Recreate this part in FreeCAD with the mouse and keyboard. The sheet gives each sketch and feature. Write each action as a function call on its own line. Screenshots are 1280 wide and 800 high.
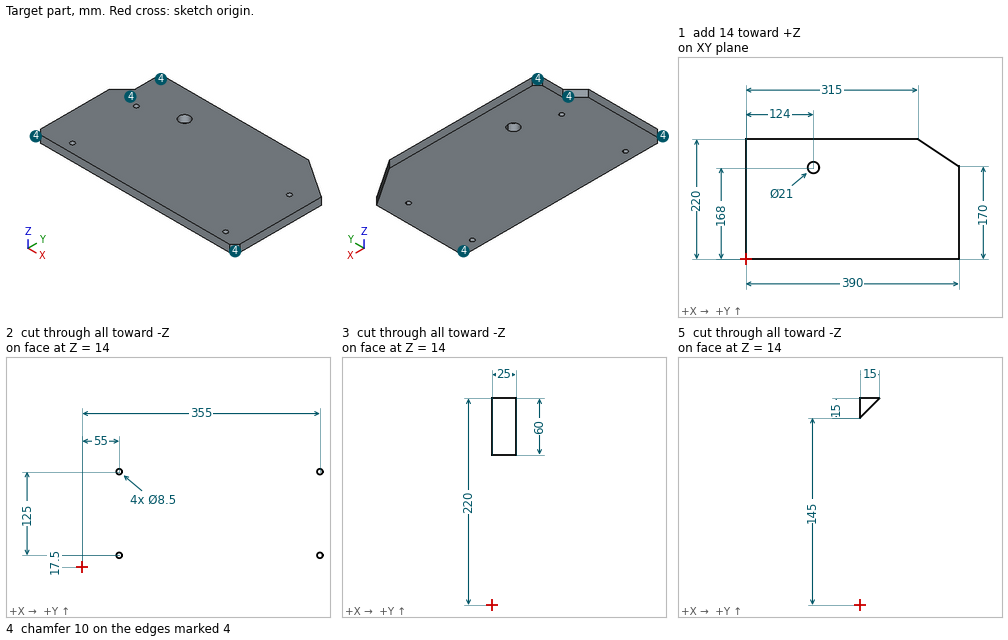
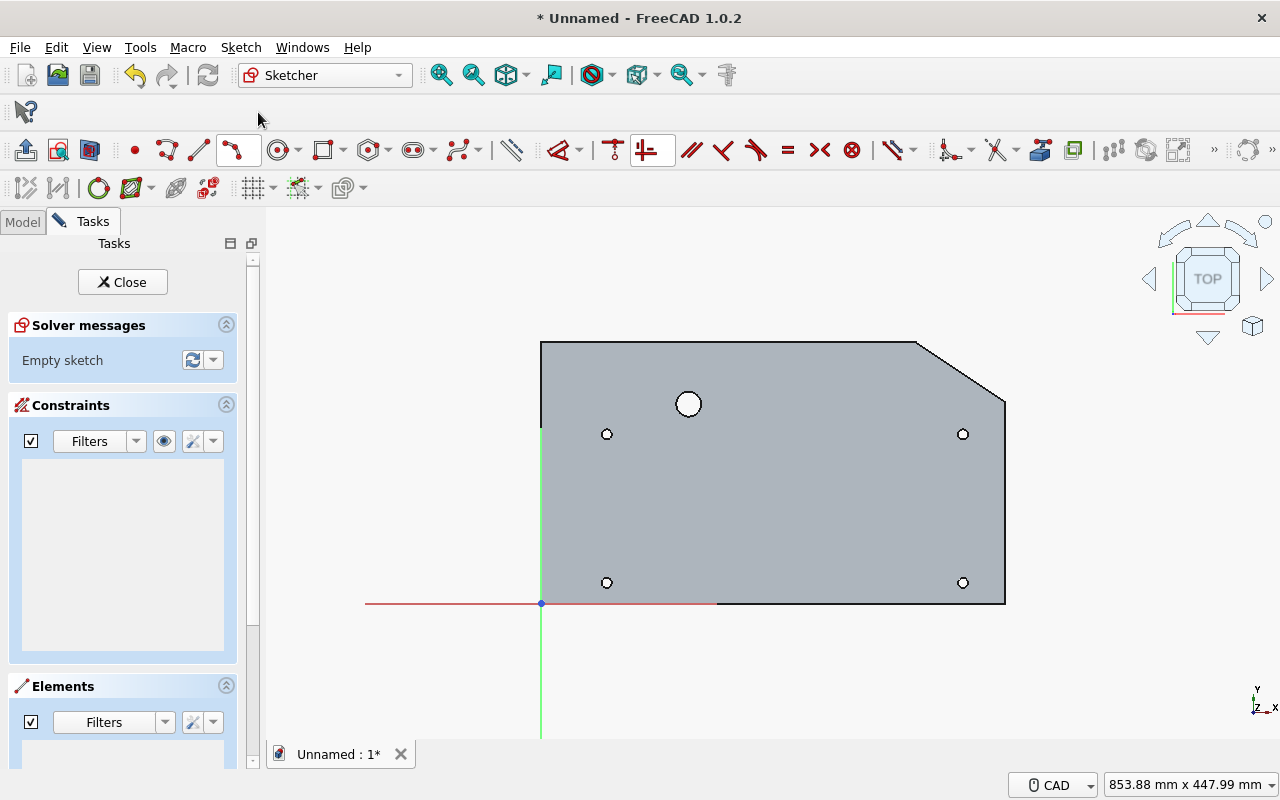
scroll(519, 354, up, 8)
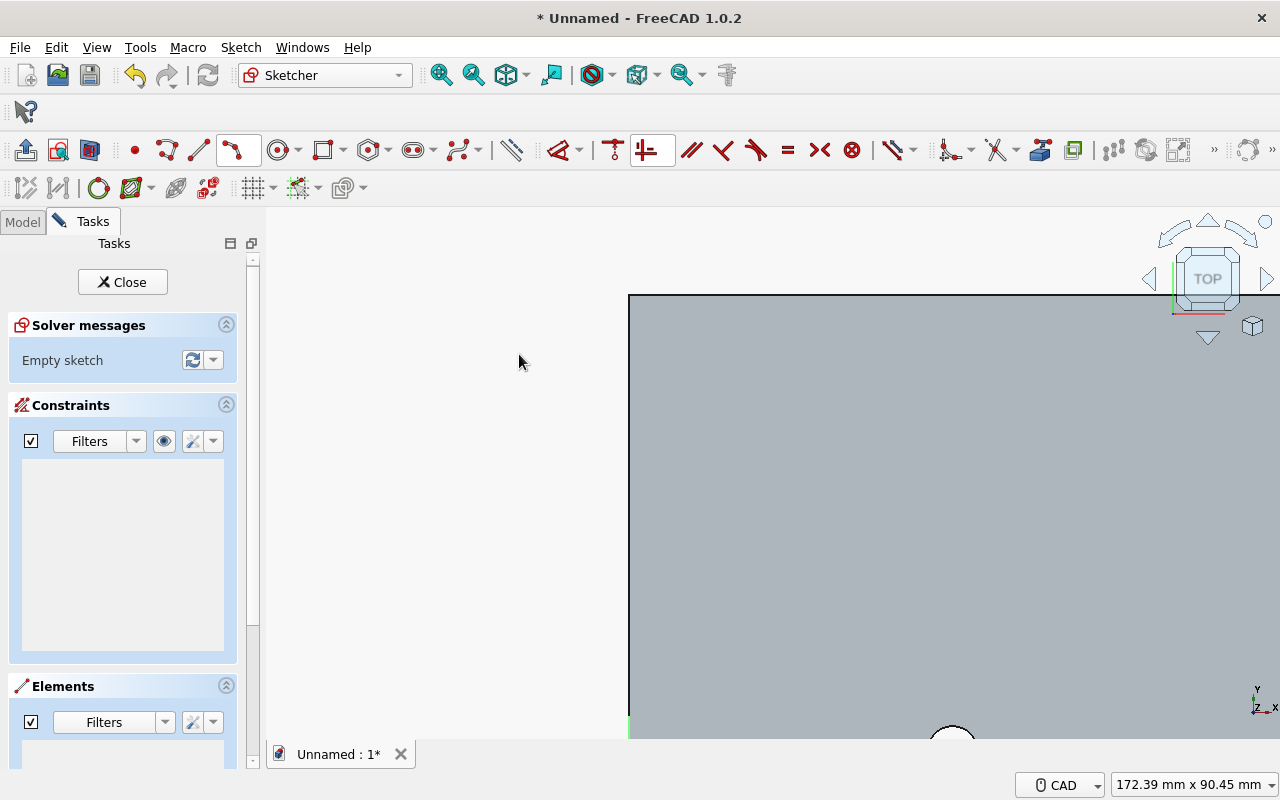
key(g)
key(r)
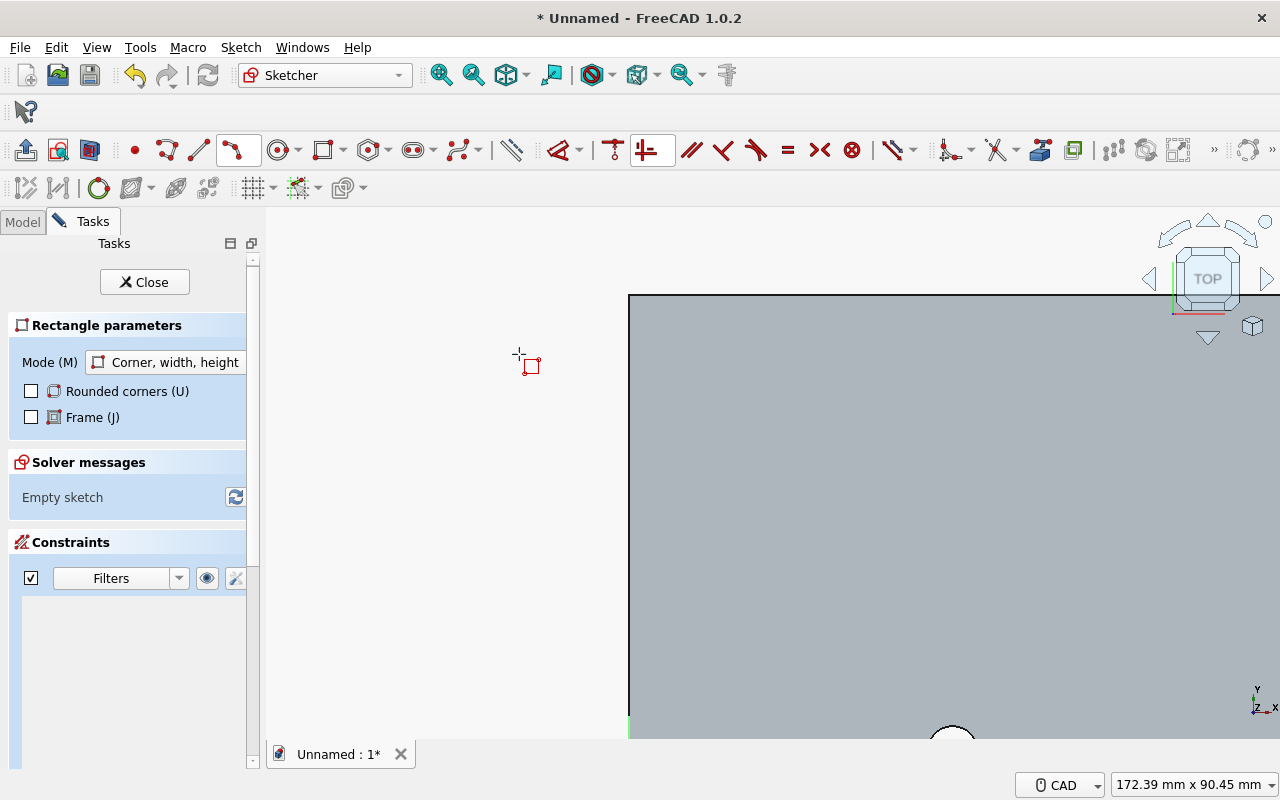
click(629, 295)
move(776, 648)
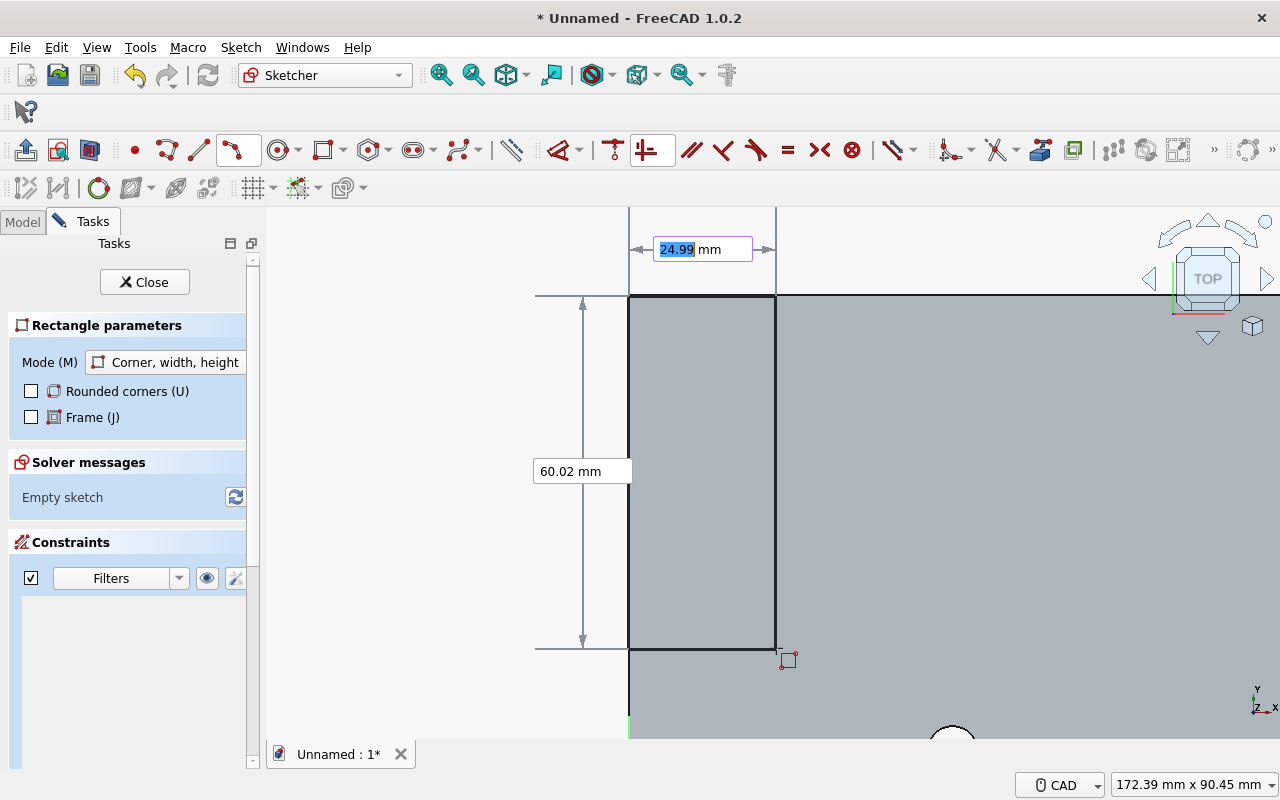
text(25)
key(Tab)
text(60)
key(Return)
key(Escape)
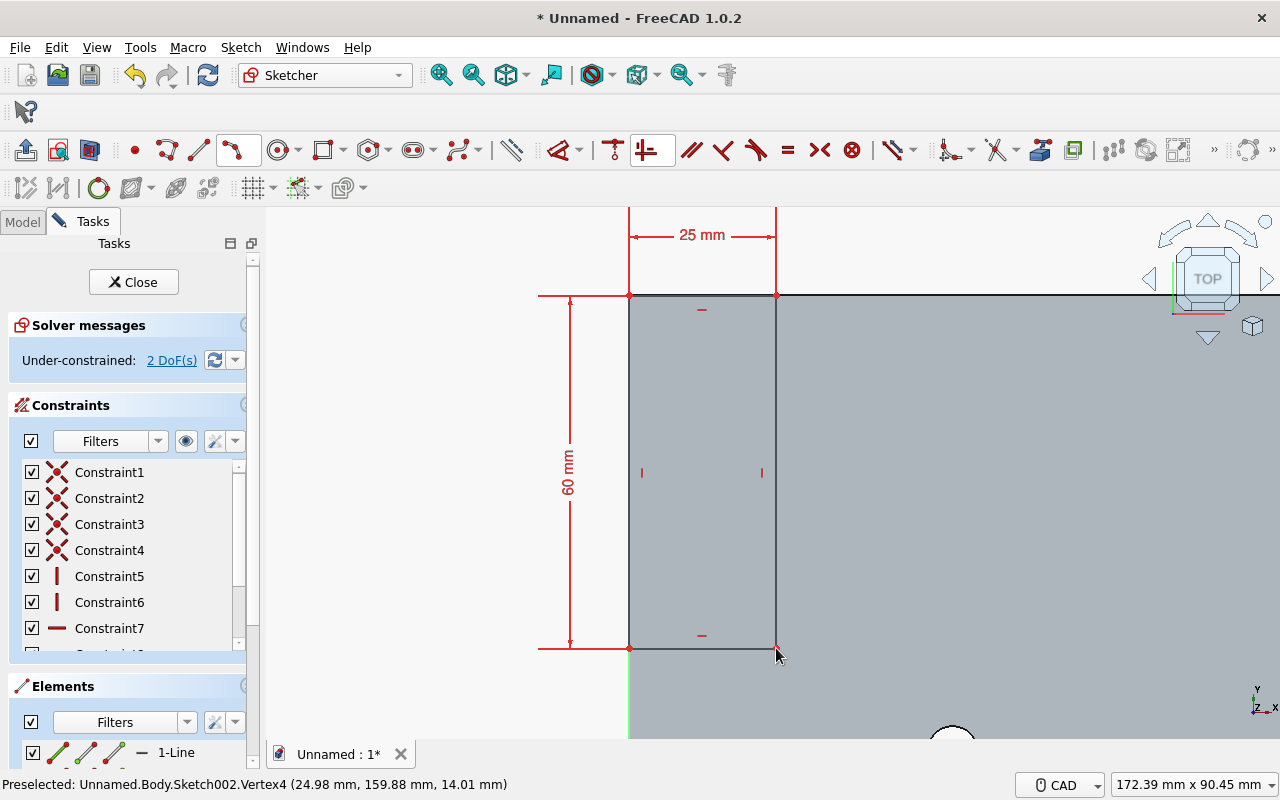
click(629, 296)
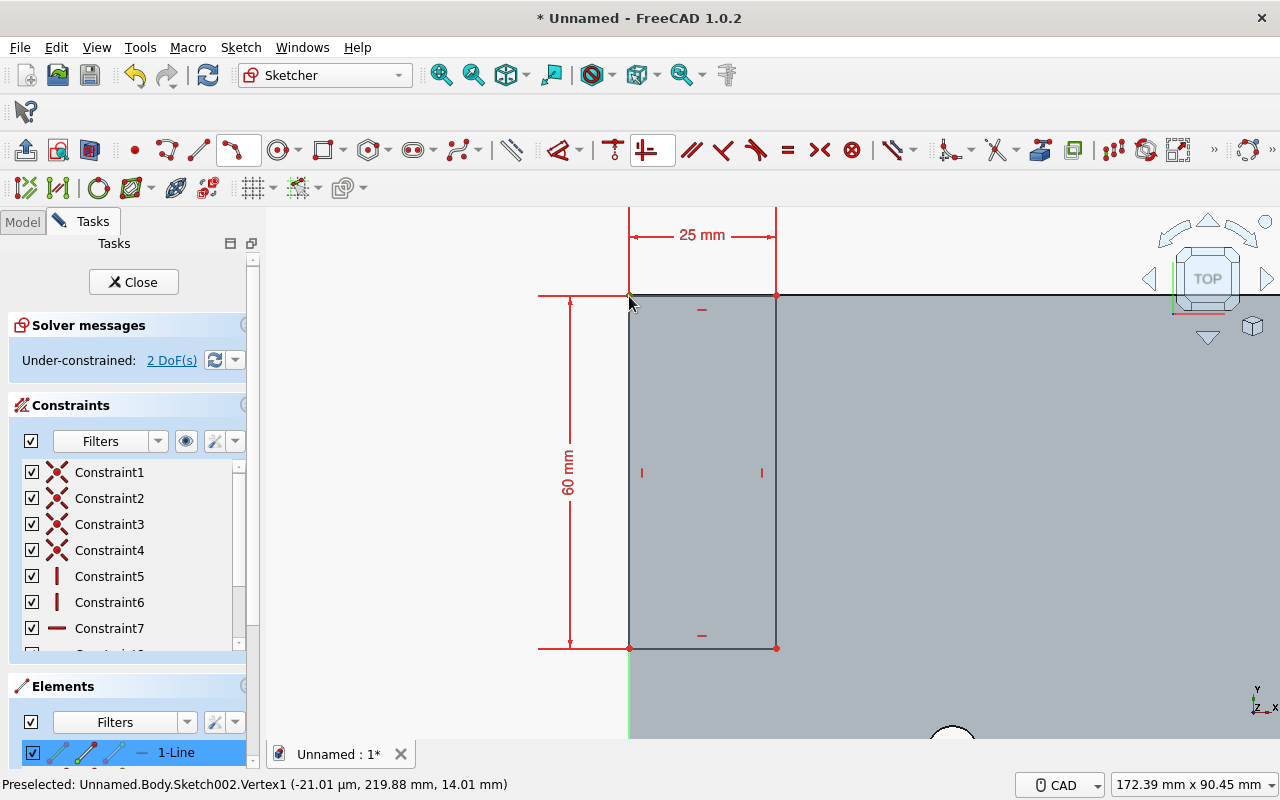
click(629, 677)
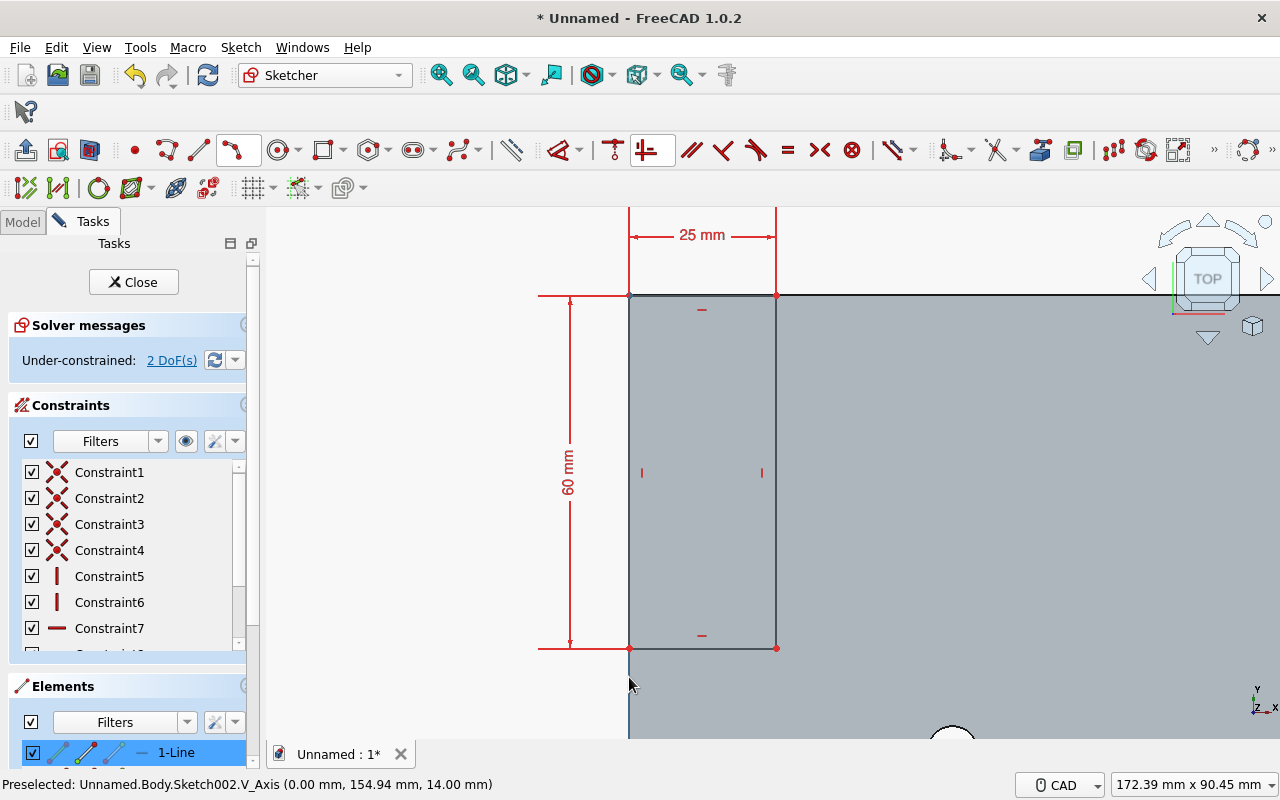
key(c)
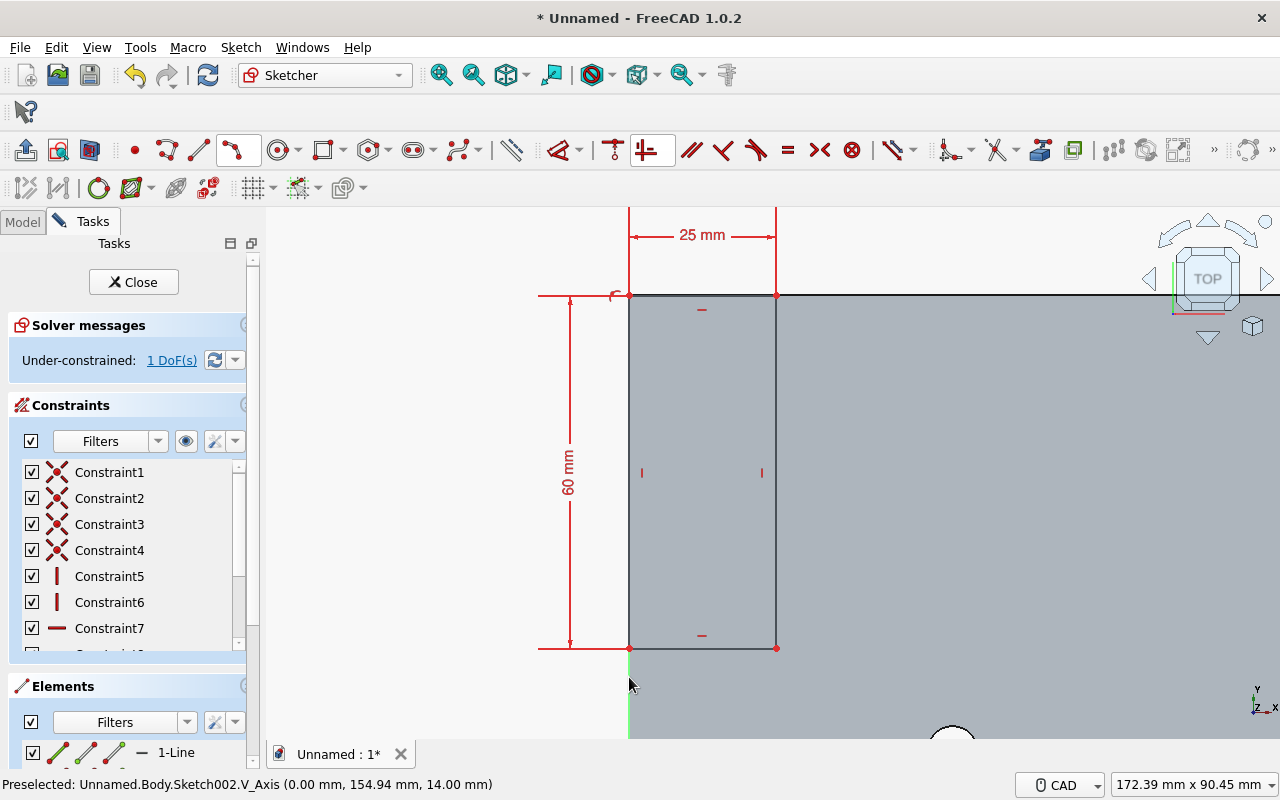
key(d)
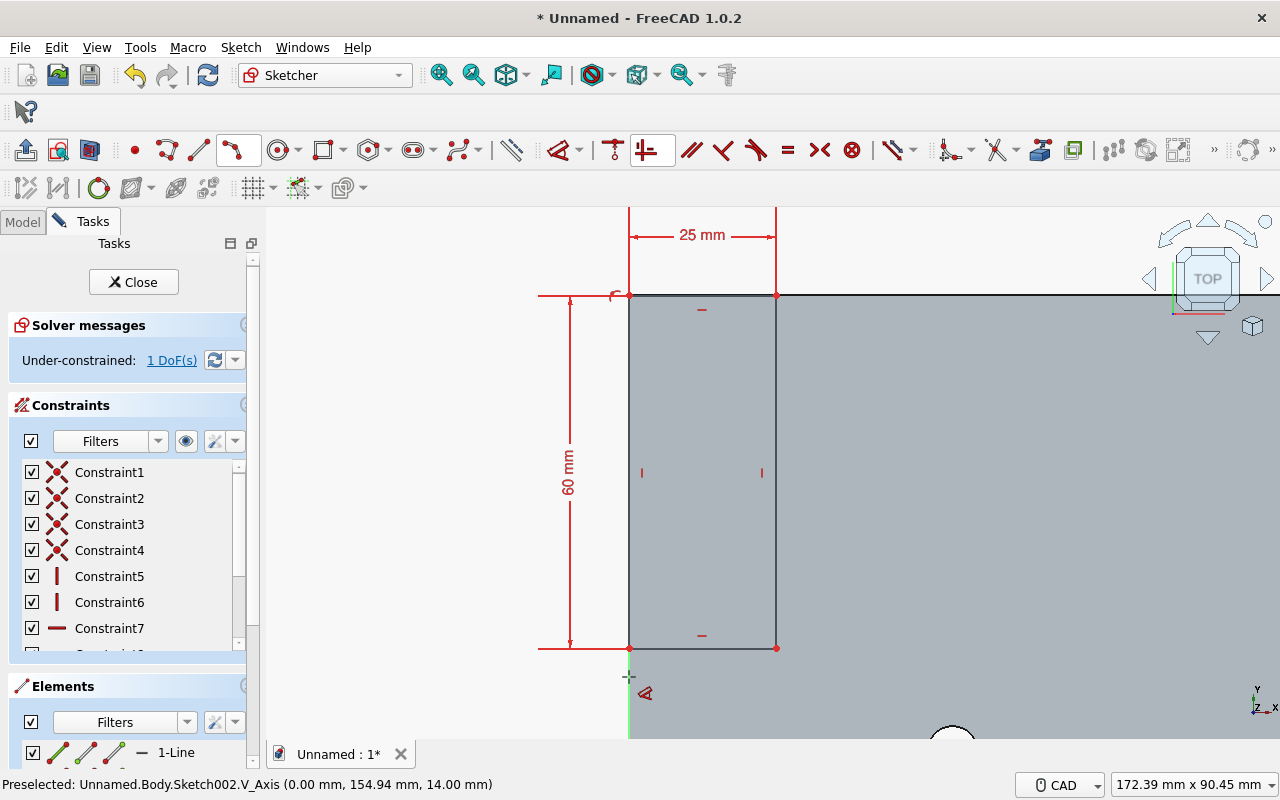
click(629, 296)
click(595, 504)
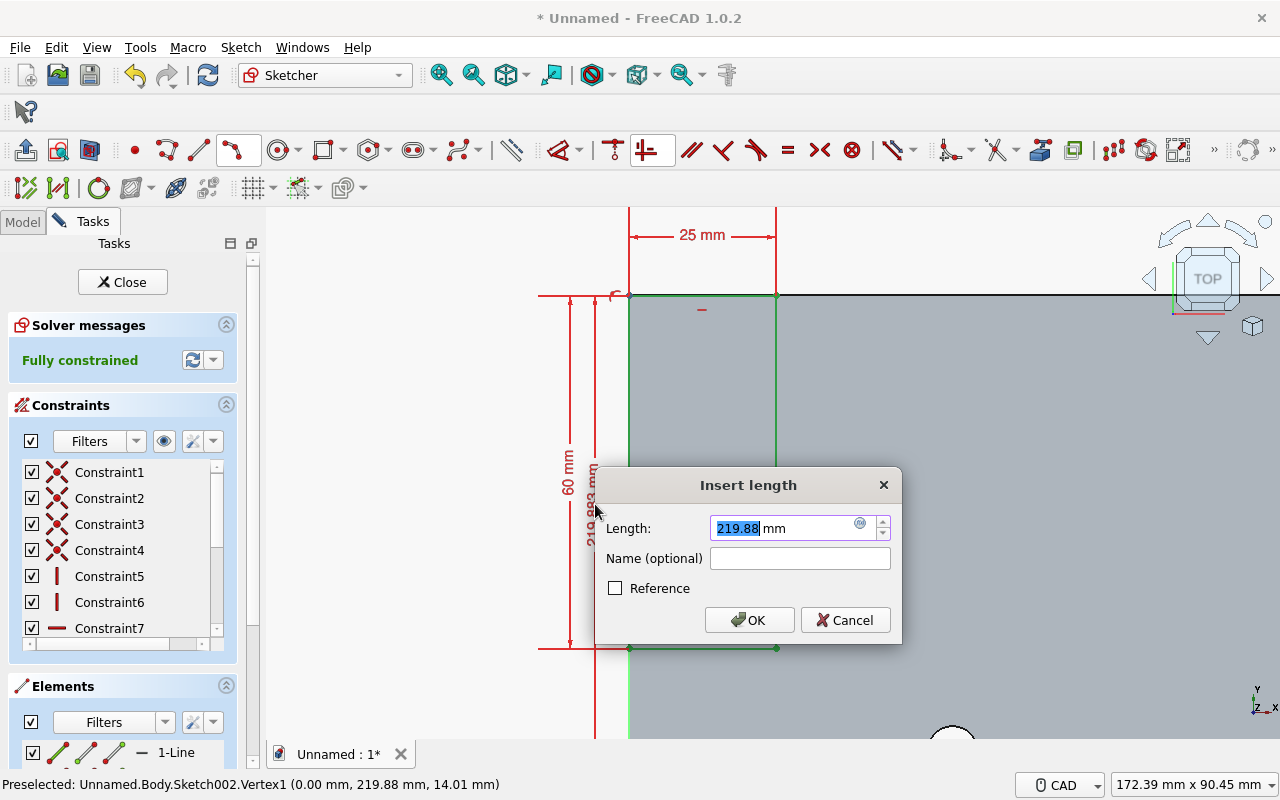
text(220)
key(Return)
key(Escape)